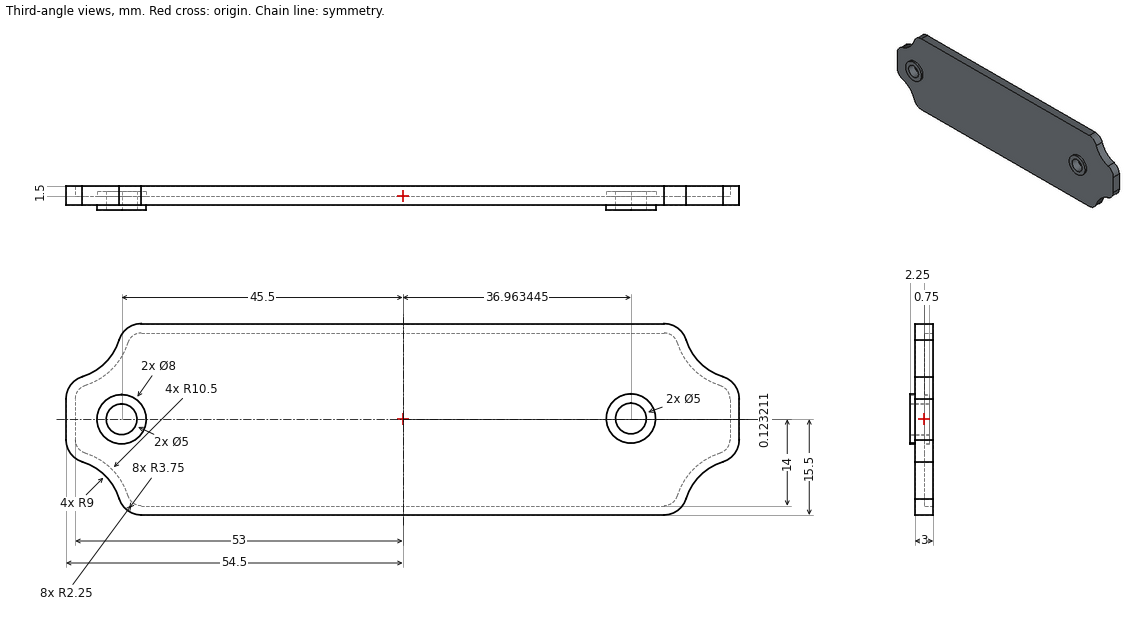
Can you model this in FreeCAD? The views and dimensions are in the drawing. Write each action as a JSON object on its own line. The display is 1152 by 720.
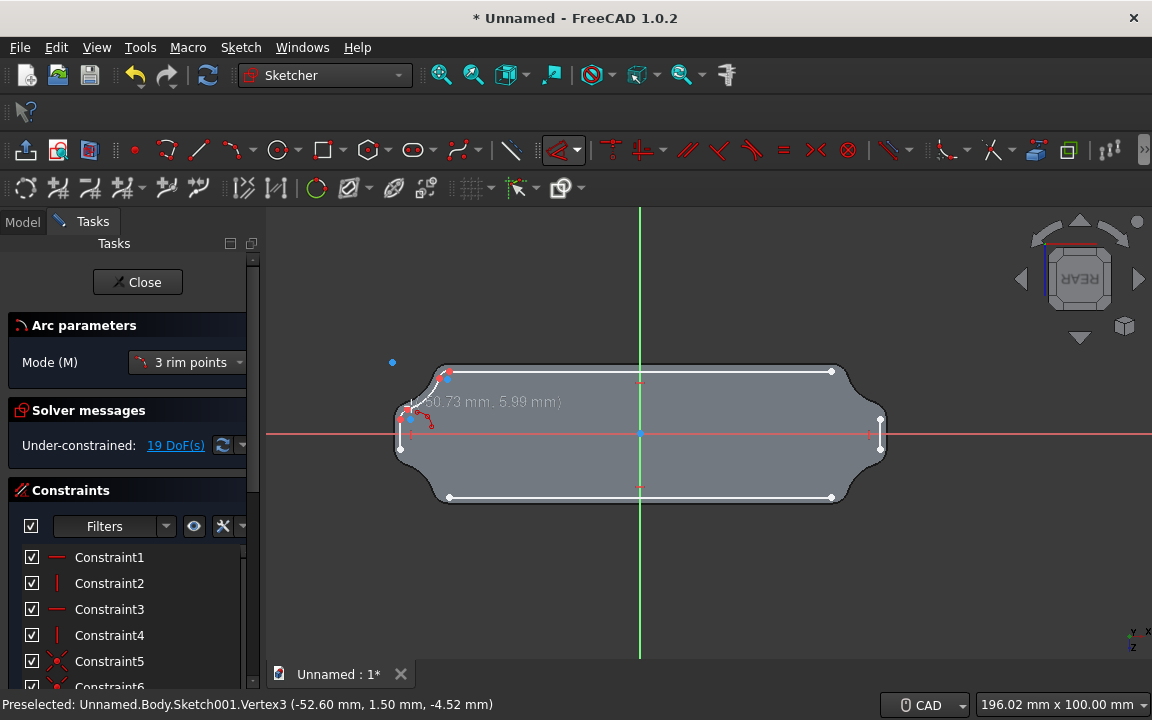
{"action": "left_click", "coordinate": [400, 450]}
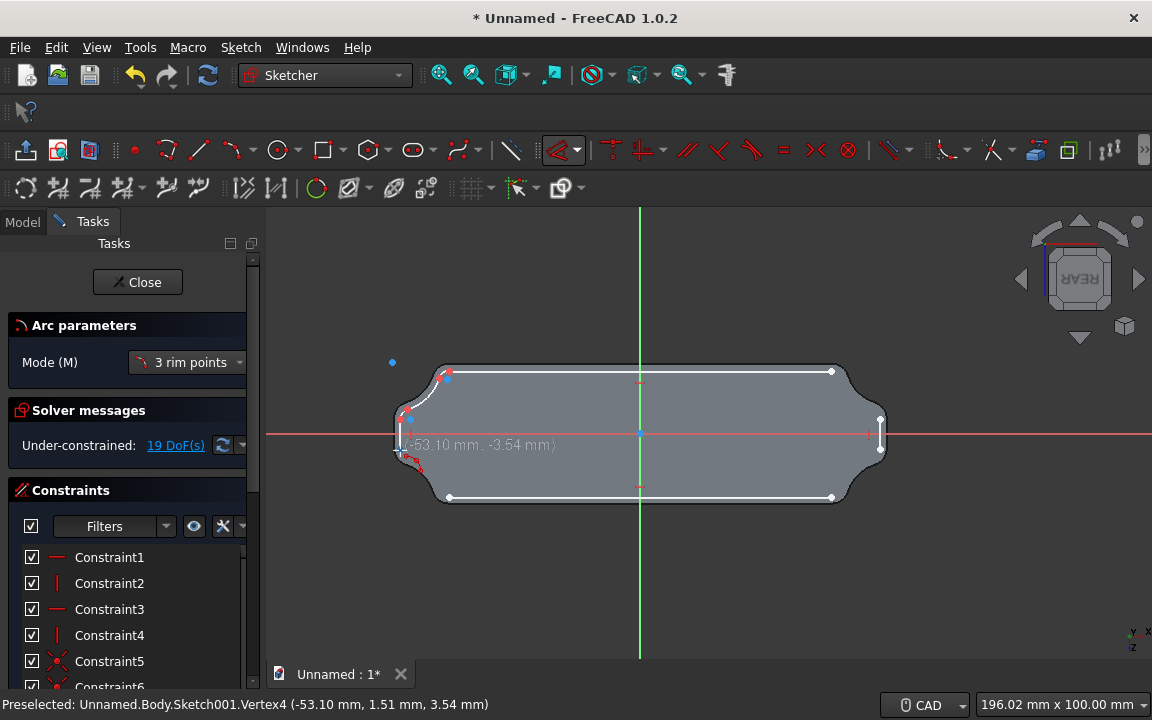
{"action": "scroll", "coordinate": [408, 458], "scroll_direction": "up", "scroll_amount": 2}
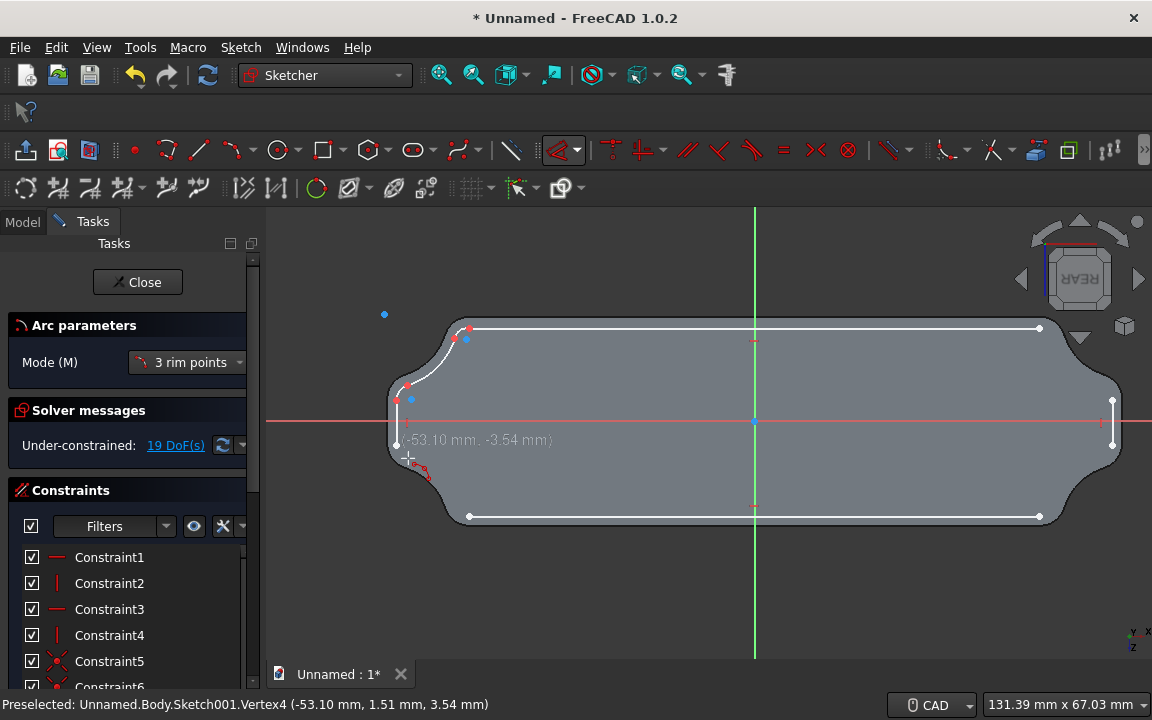
{"action": "left_click", "coordinate": [408, 458]}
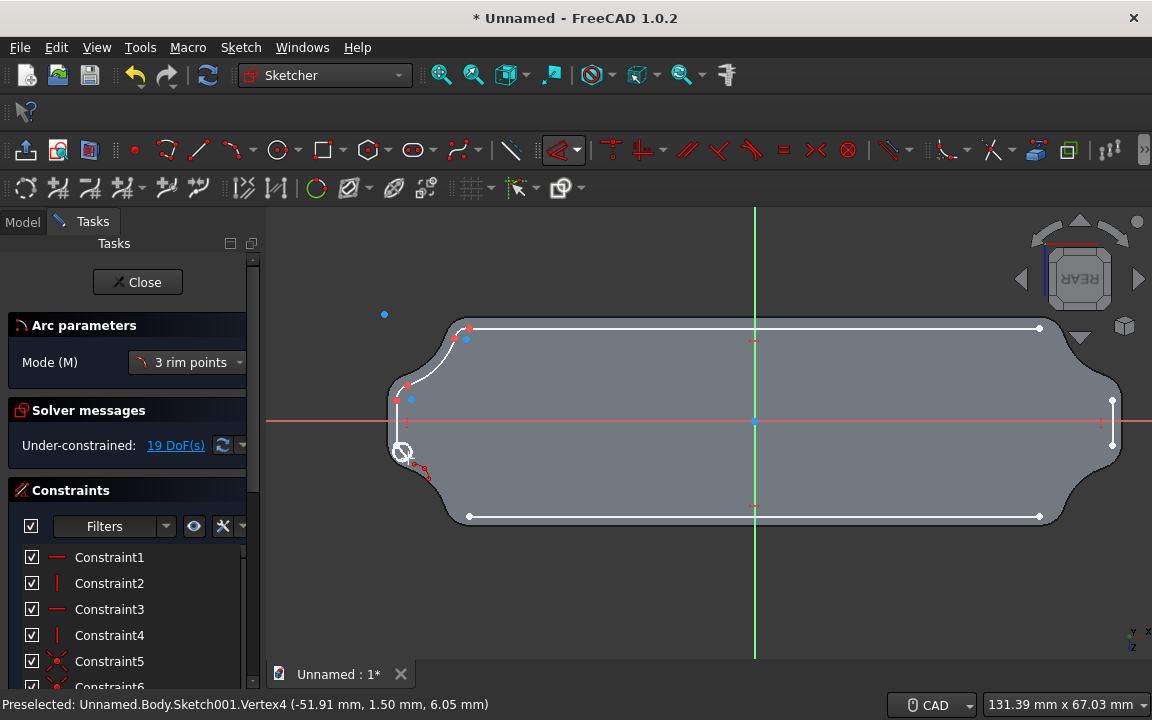
{"action": "scroll", "coordinate": [400, 453], "scroll_direction": "up", "scroll_amount": 9}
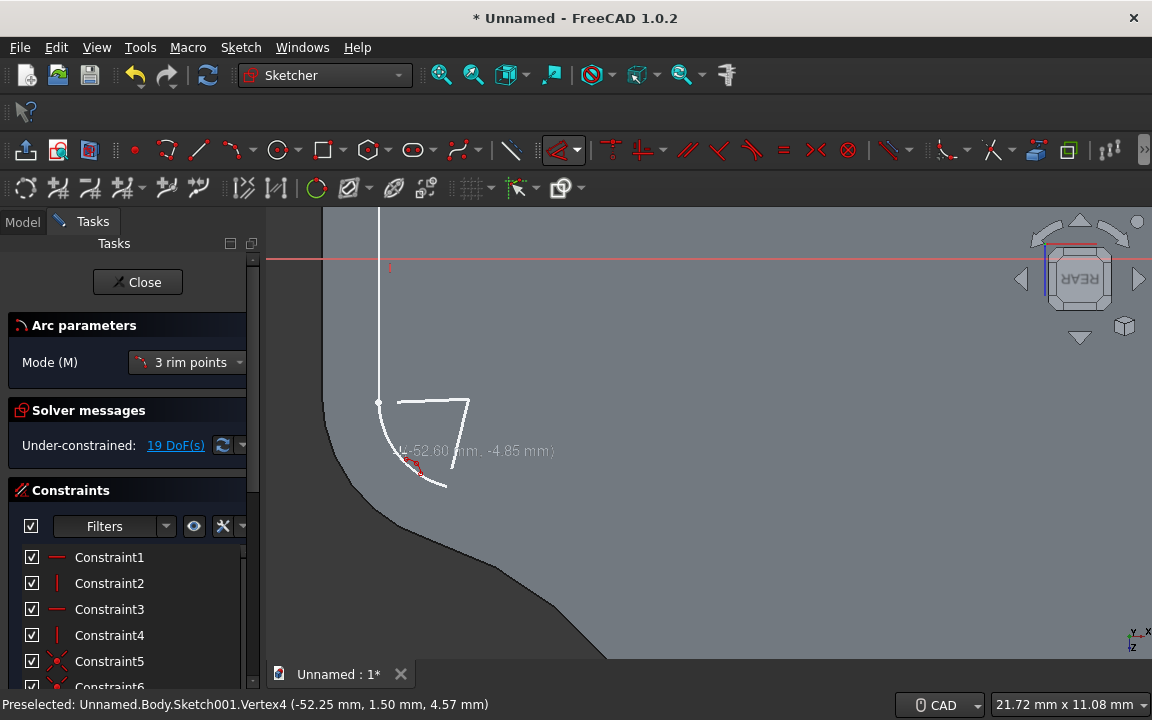
{"action": "left_click", "coordinate": [401, 448]}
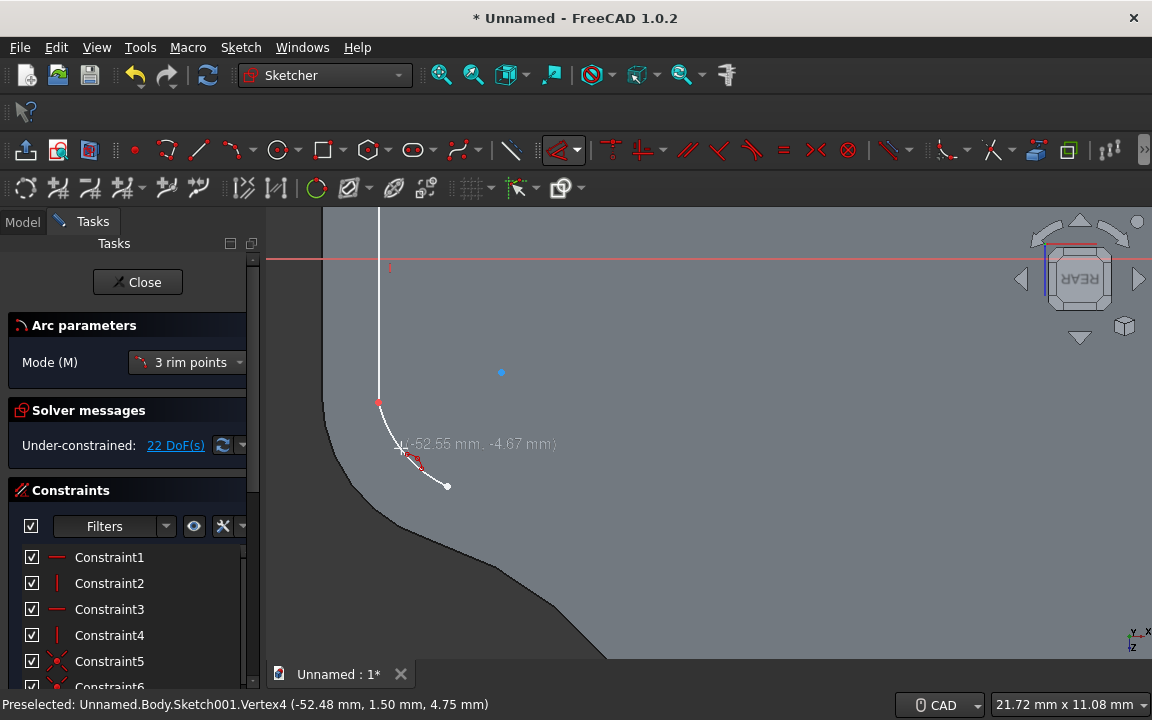
{"action": "scroll", "coordinate": [403, 455], "scroll_direction": "down", "scroll_amount": 11}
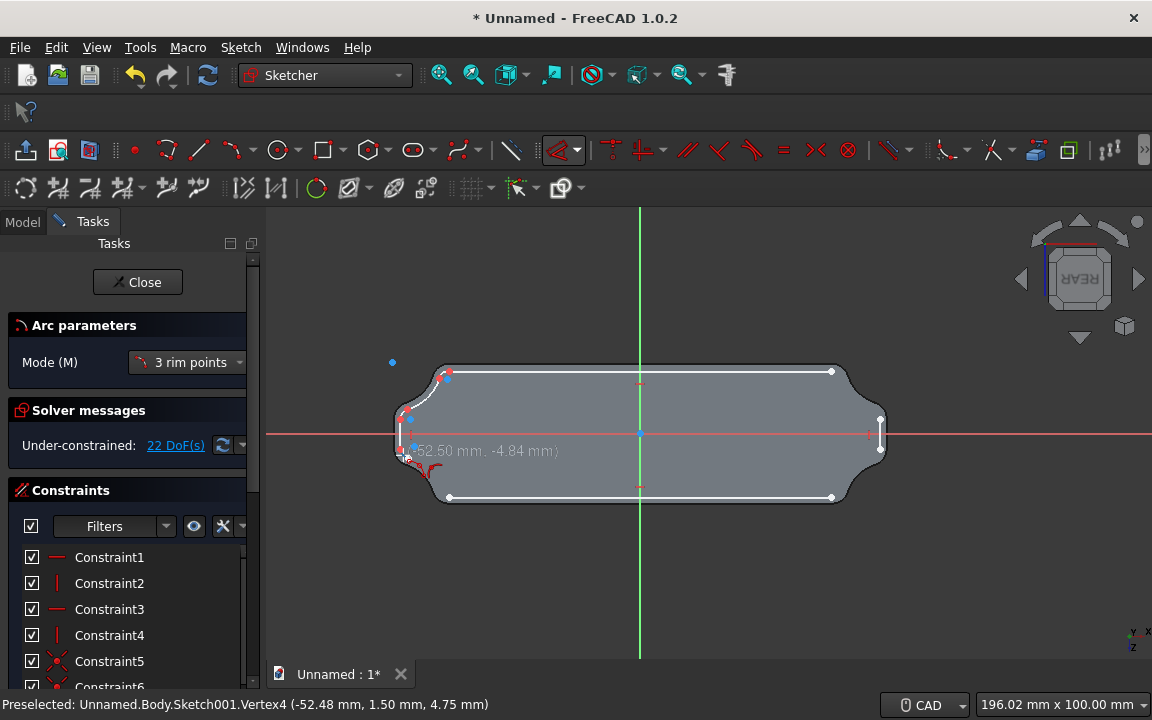
{"action": "scroll", "coordinate": [408, 458], "scroll_direction": "up", "scroll_amount": 3}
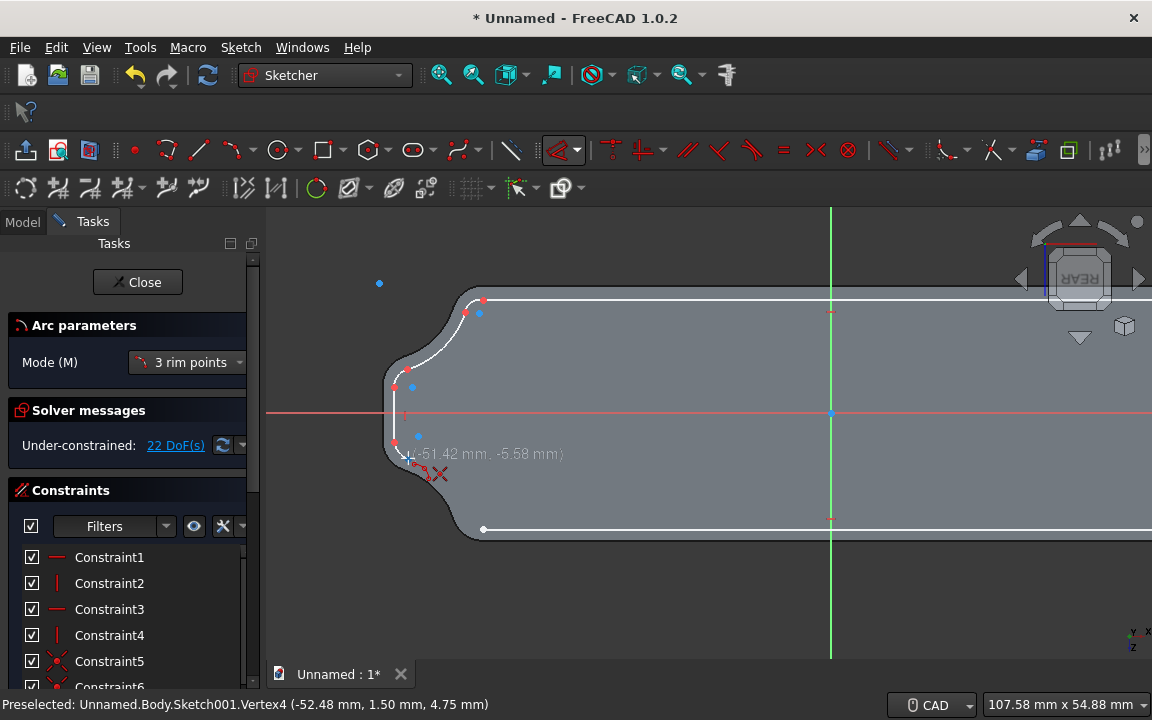
{"action": "left_click", "coordinate": [408, 459]}
{"action": "left_click", "coordinate": [465, 516]}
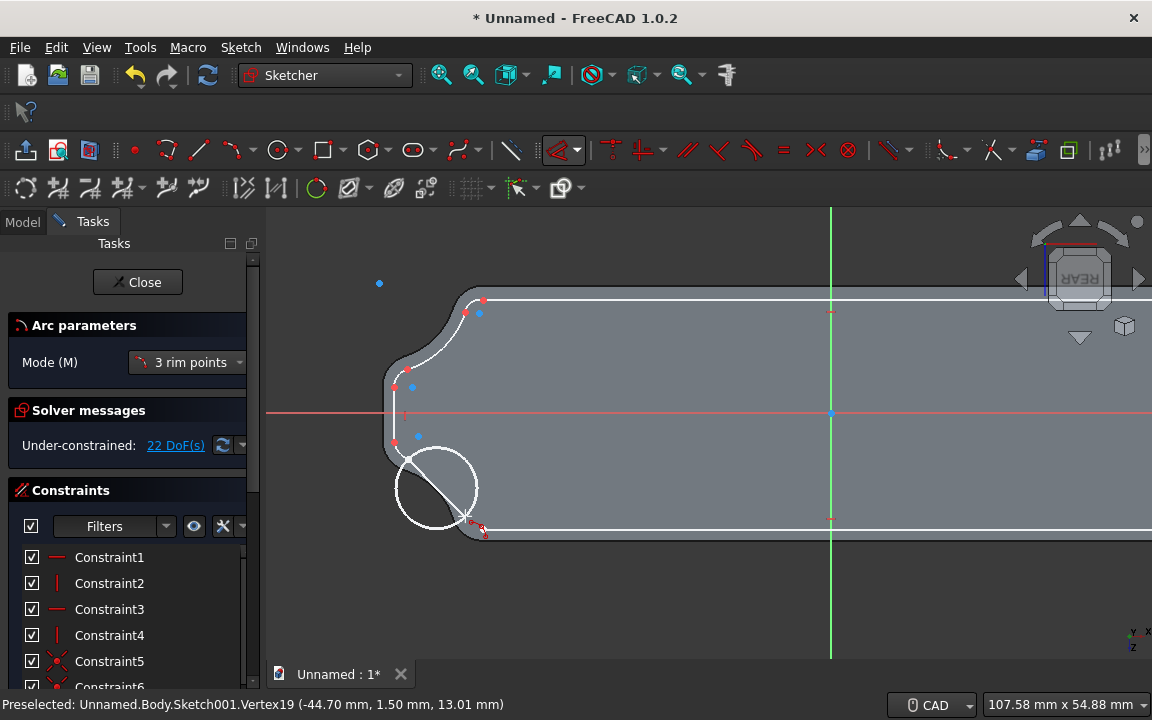
{"action": "scroll", "coordinate": [444, 480], "scroll_direction": "up", "scroll_amount": 3}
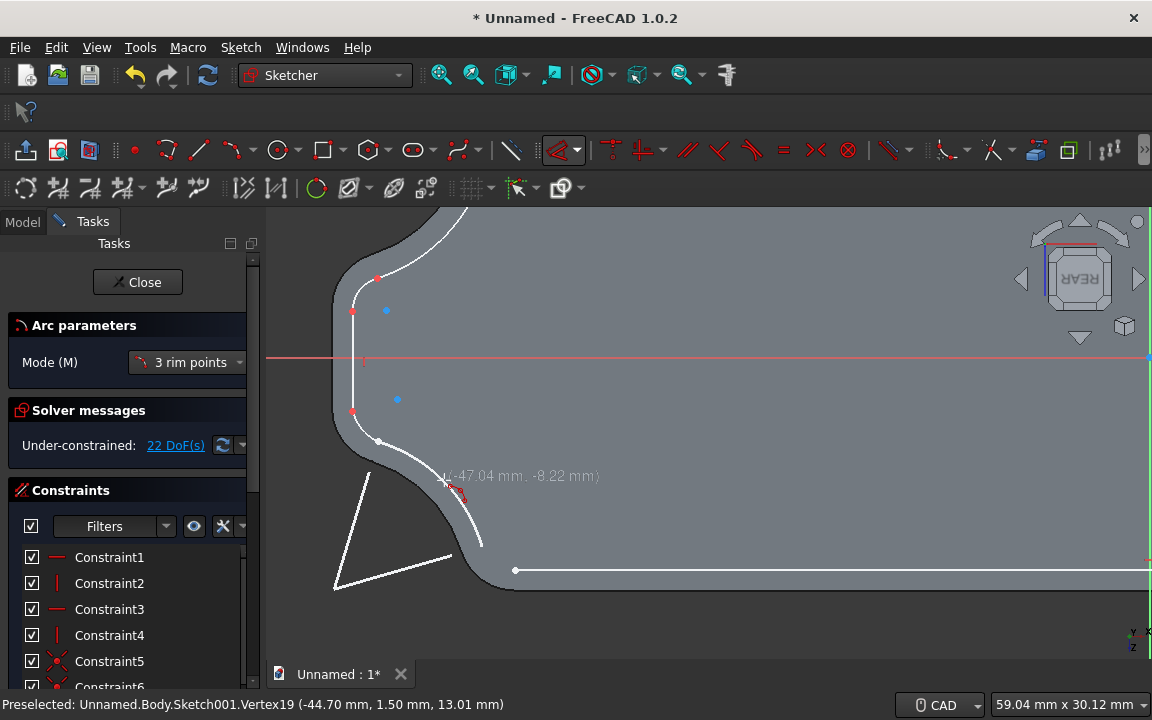
{"action": "left_click", "coordinate": [443, 479]}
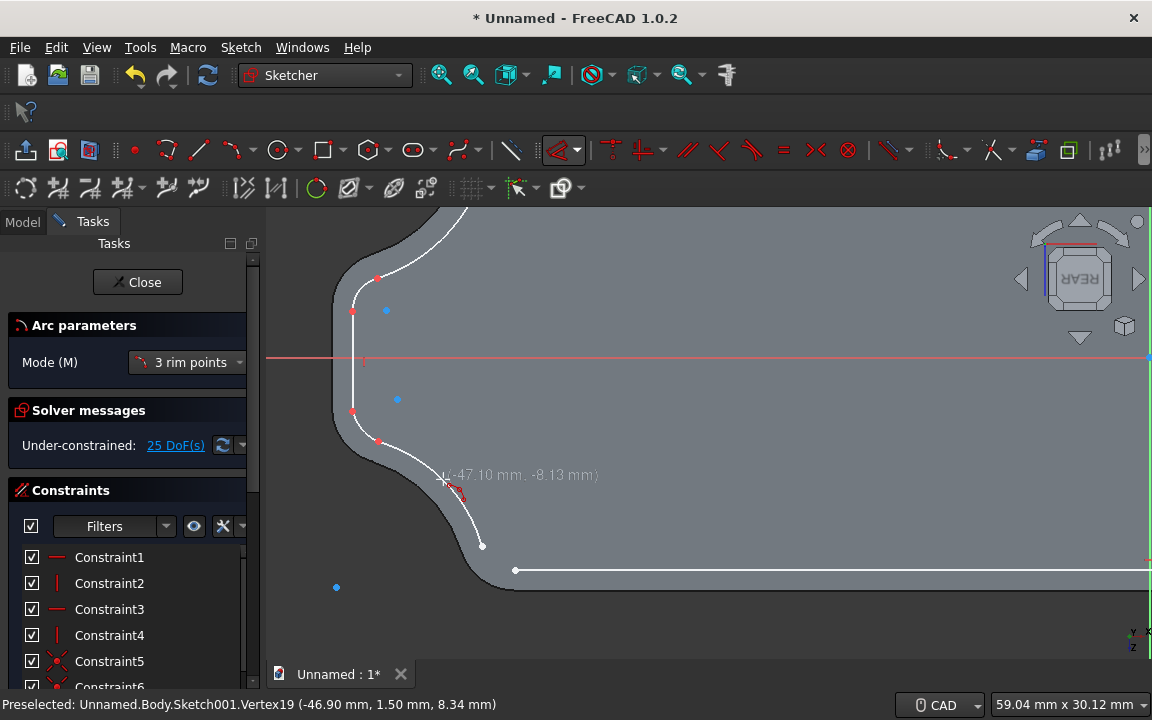
{"action": "left_click", "coordinate": [482, 547]}
{"action": "left_click", "coordinate": [516, 570]}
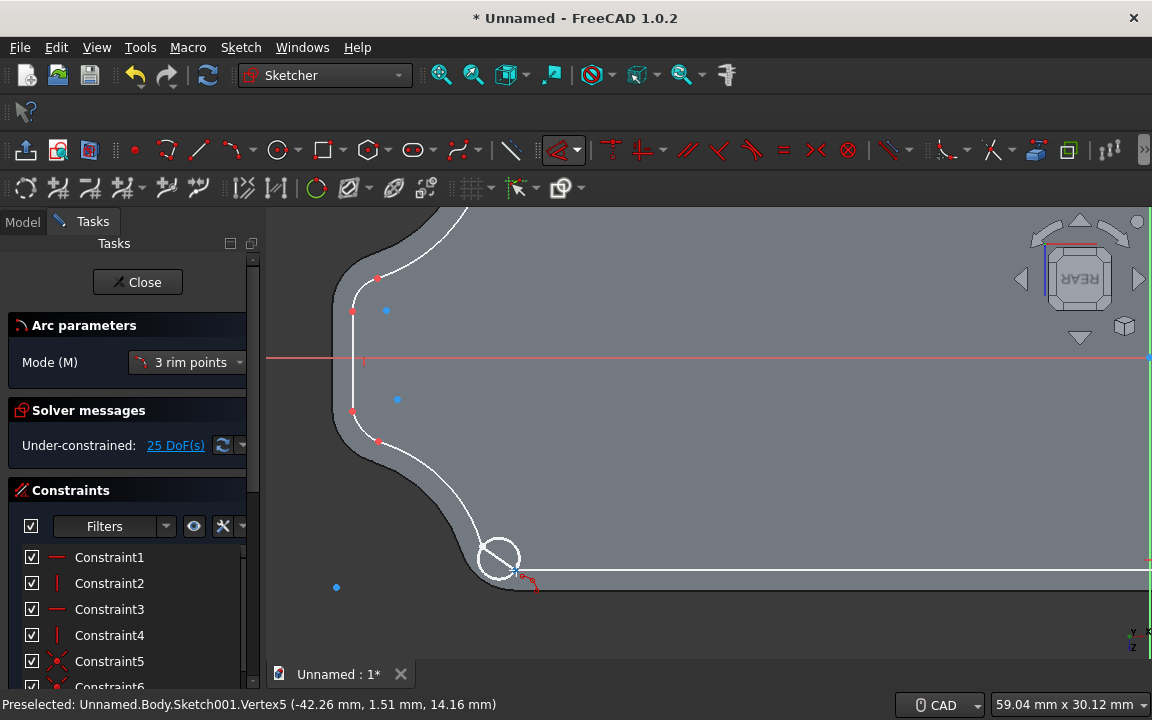
{"action": "scroll", "coordinate": [495, 561], "scroll_direction": "up", "scroll_amount": 5}